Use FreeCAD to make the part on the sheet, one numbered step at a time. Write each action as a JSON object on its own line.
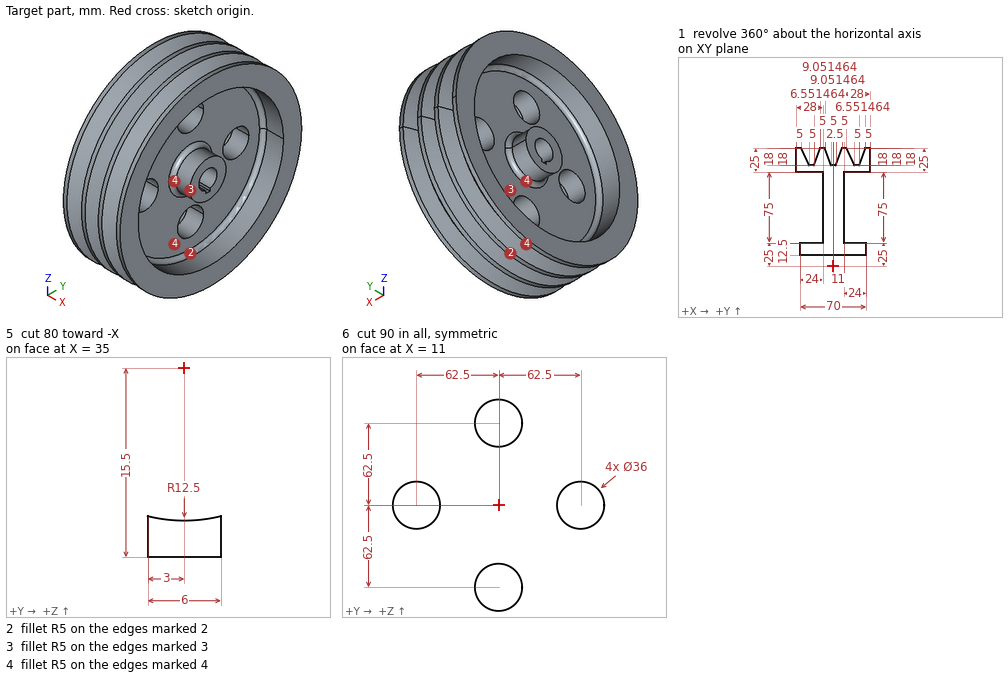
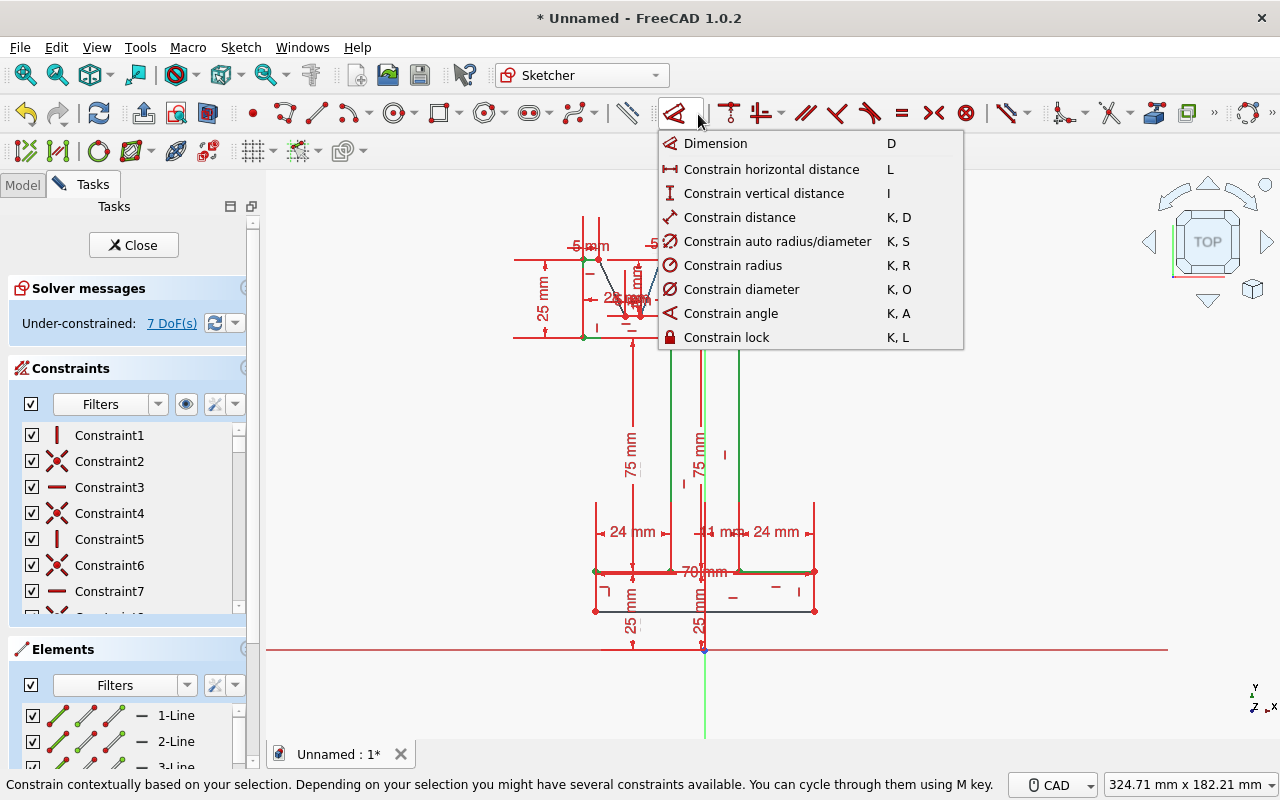
{"action": "left_click", "coordinate": [811, 193]}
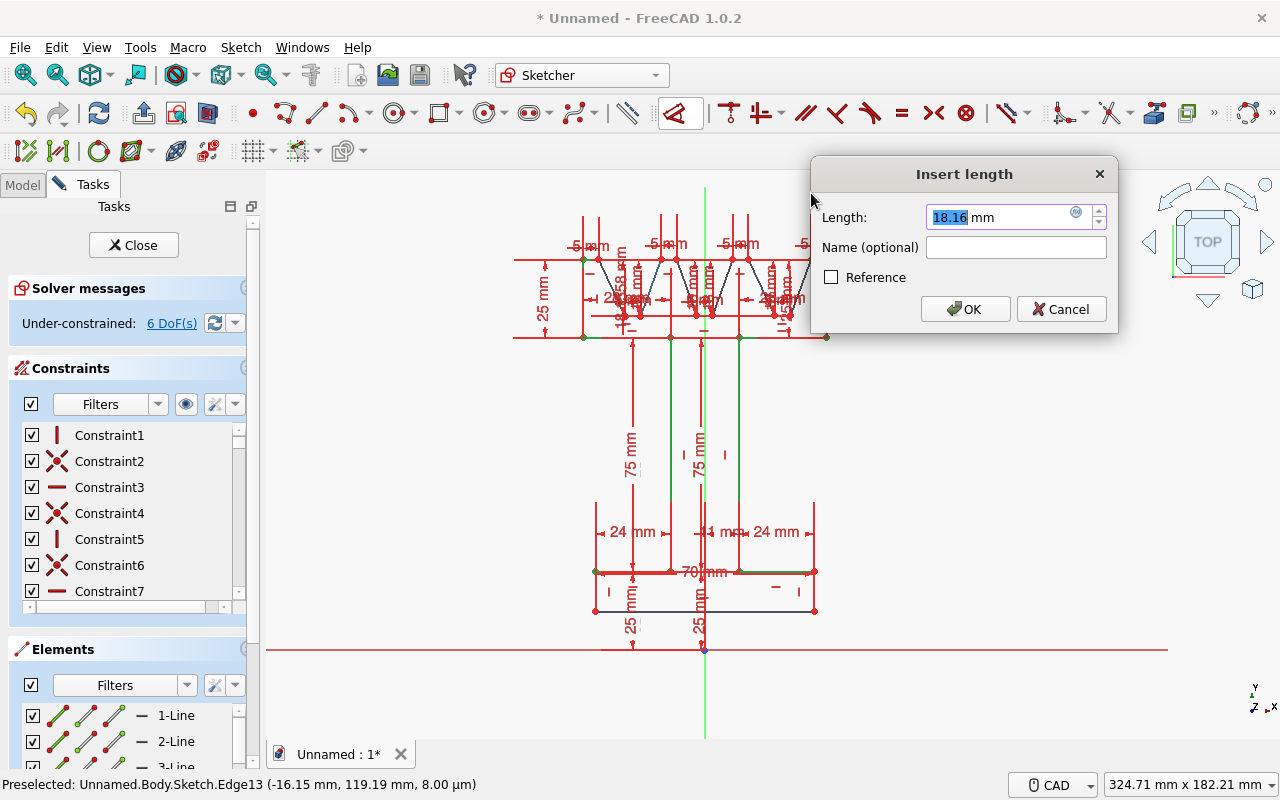
{"action": "type", "text": "18"}
{"action": "key", "text": "Return"}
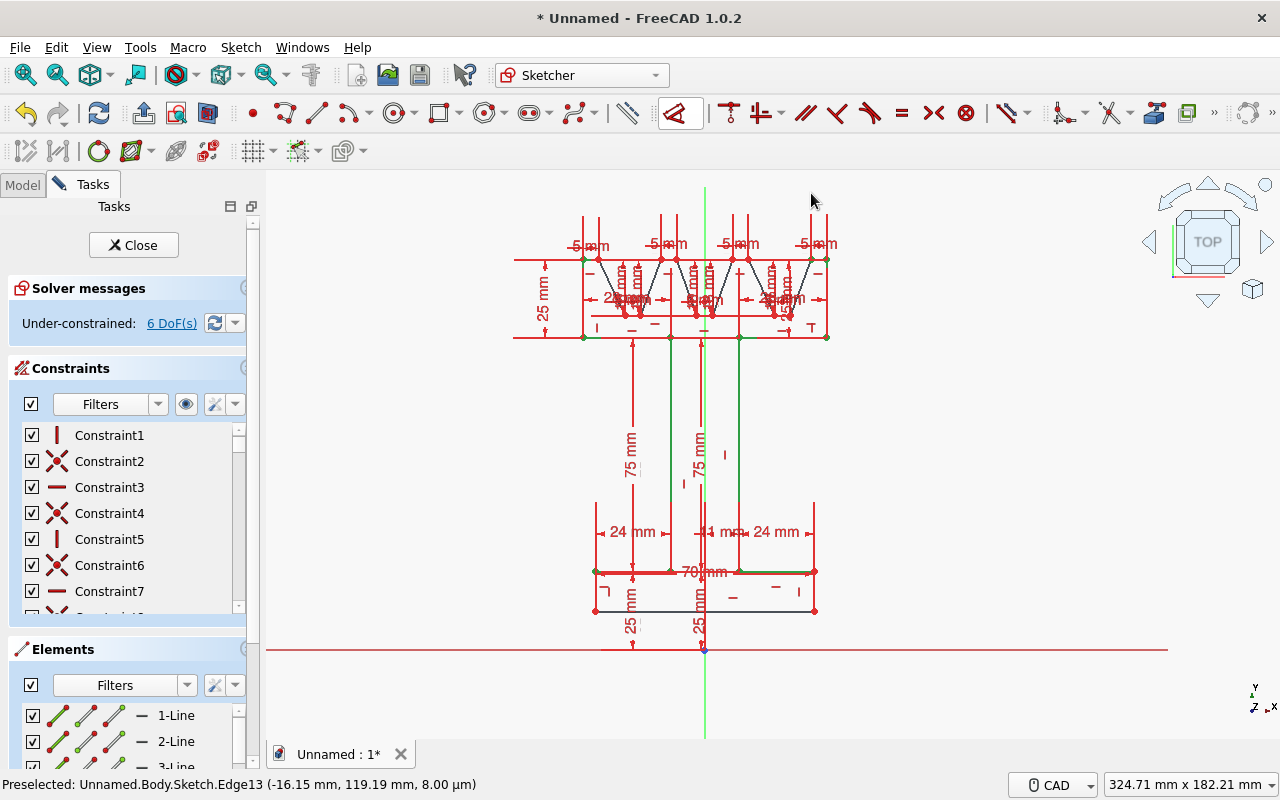
{"action": "left_click", "coordinate": [596, 584]}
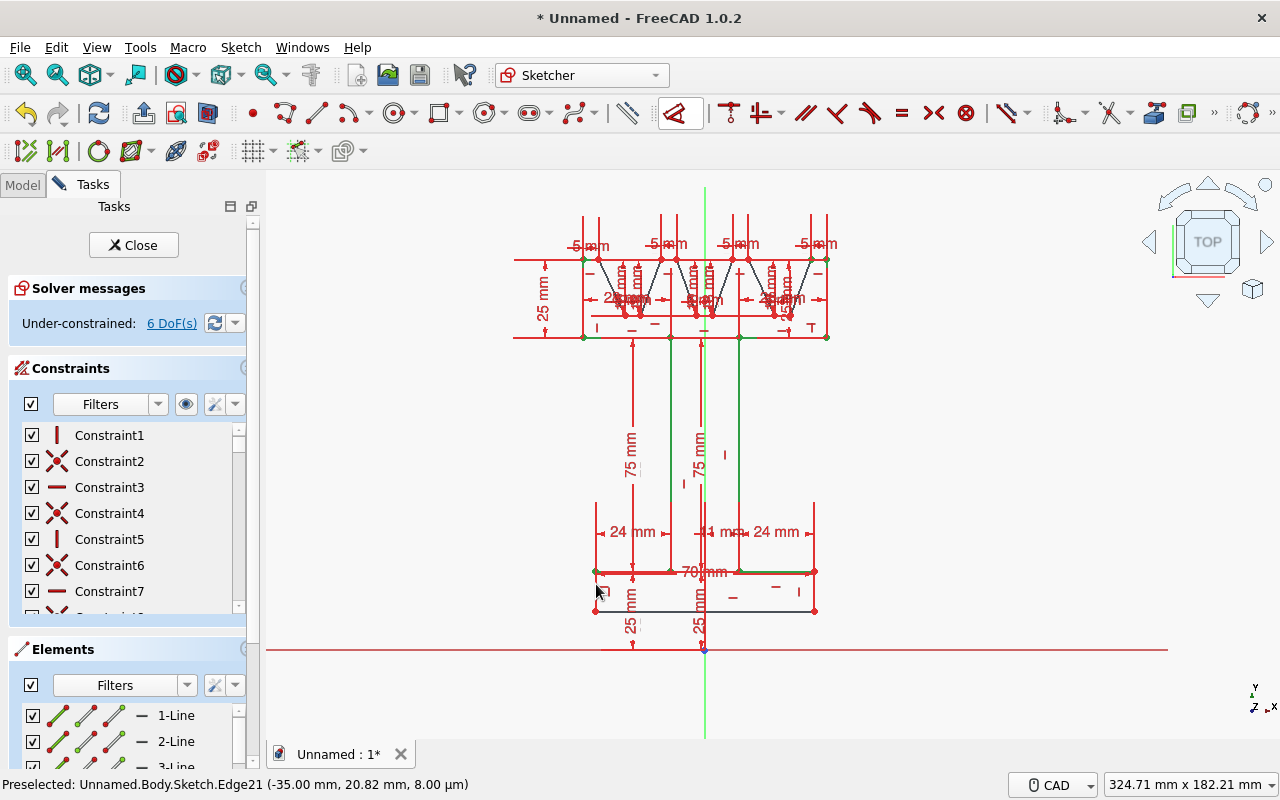
{"action": "key", "text": "i"}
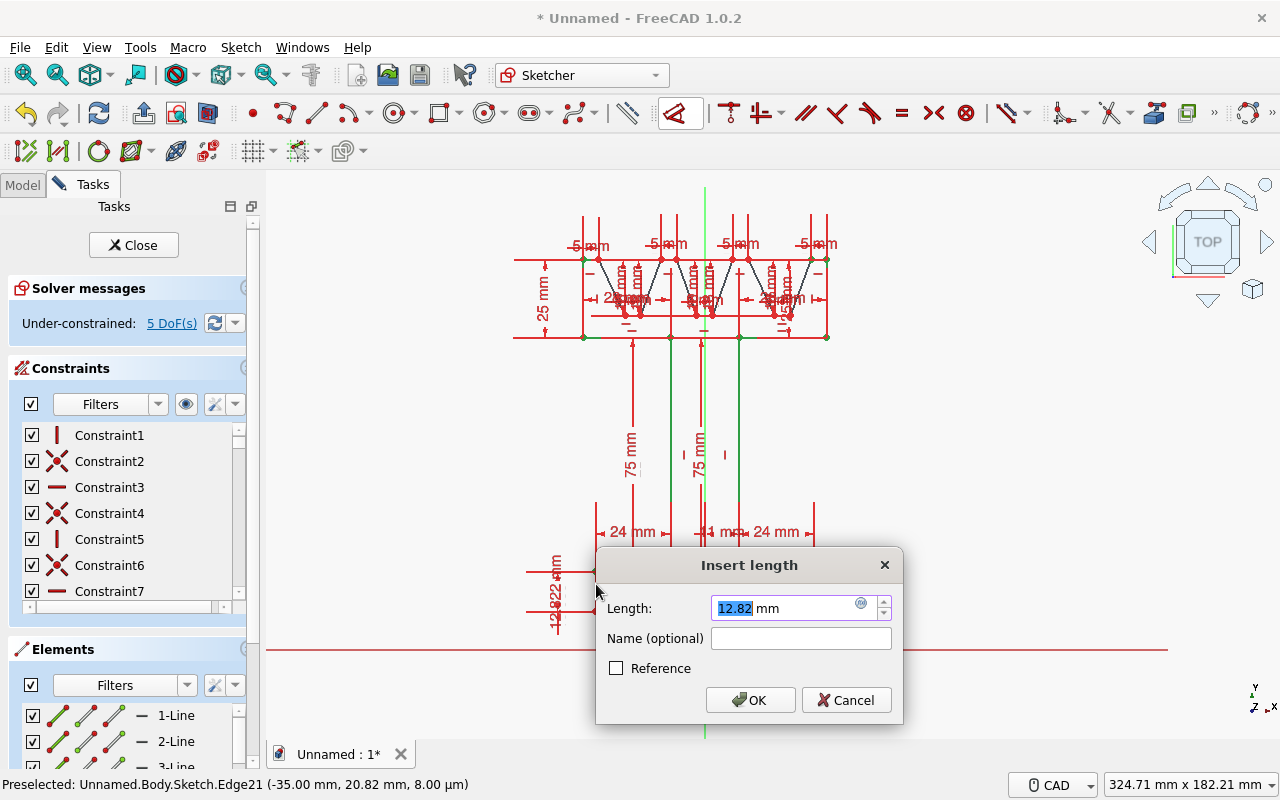
{"action": "type", "text": "12.5"}
{"action": "key", "text": "Return"}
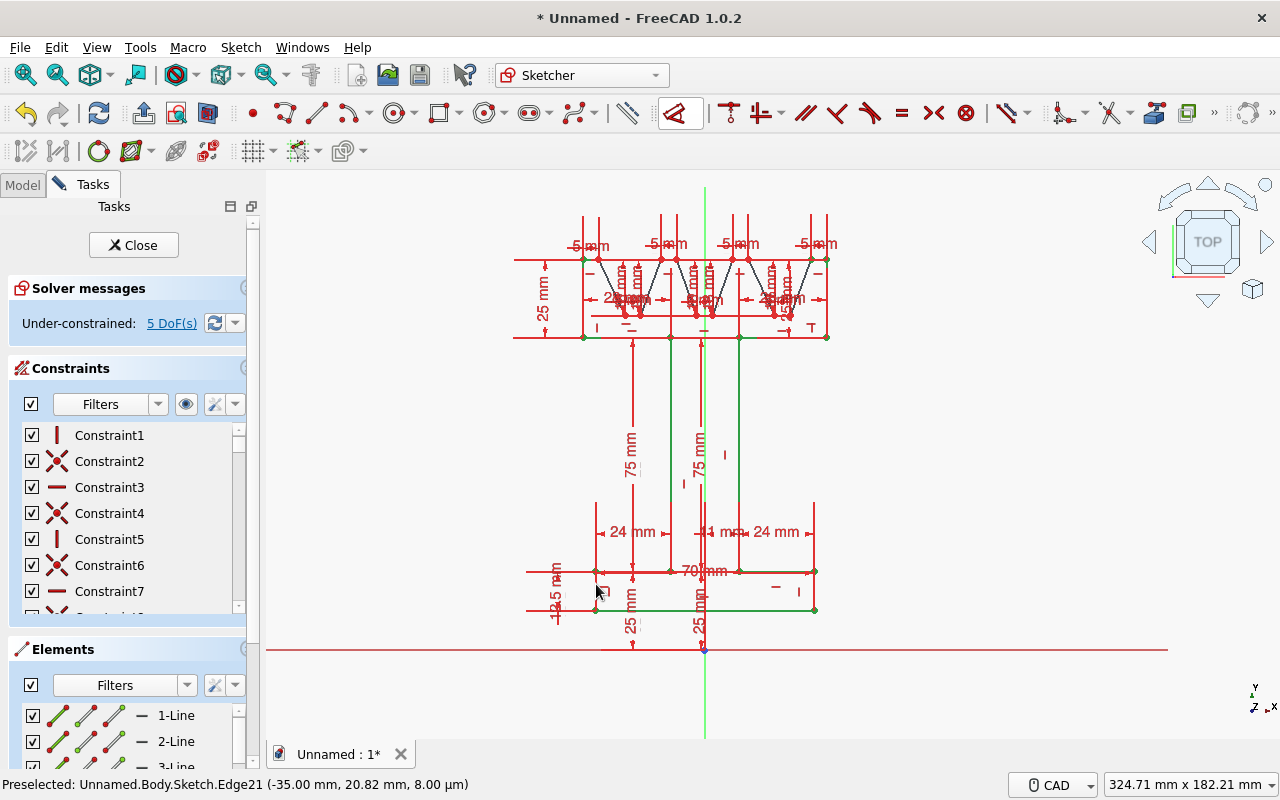
{"action": "scroll", "coordinate": [713, 316], "scroll_direction": "up", "scroll_amount": 9}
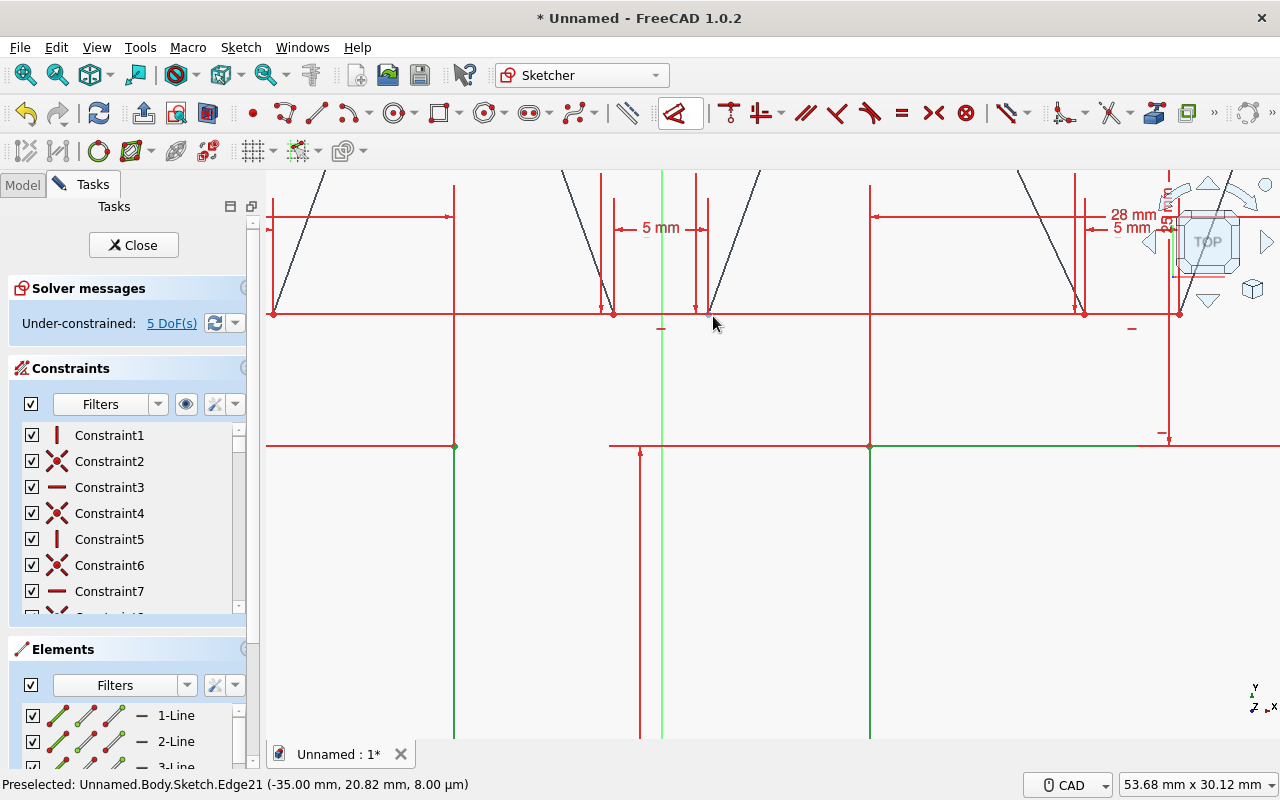
{"action": "left_click", "coordinate": [708, 314]}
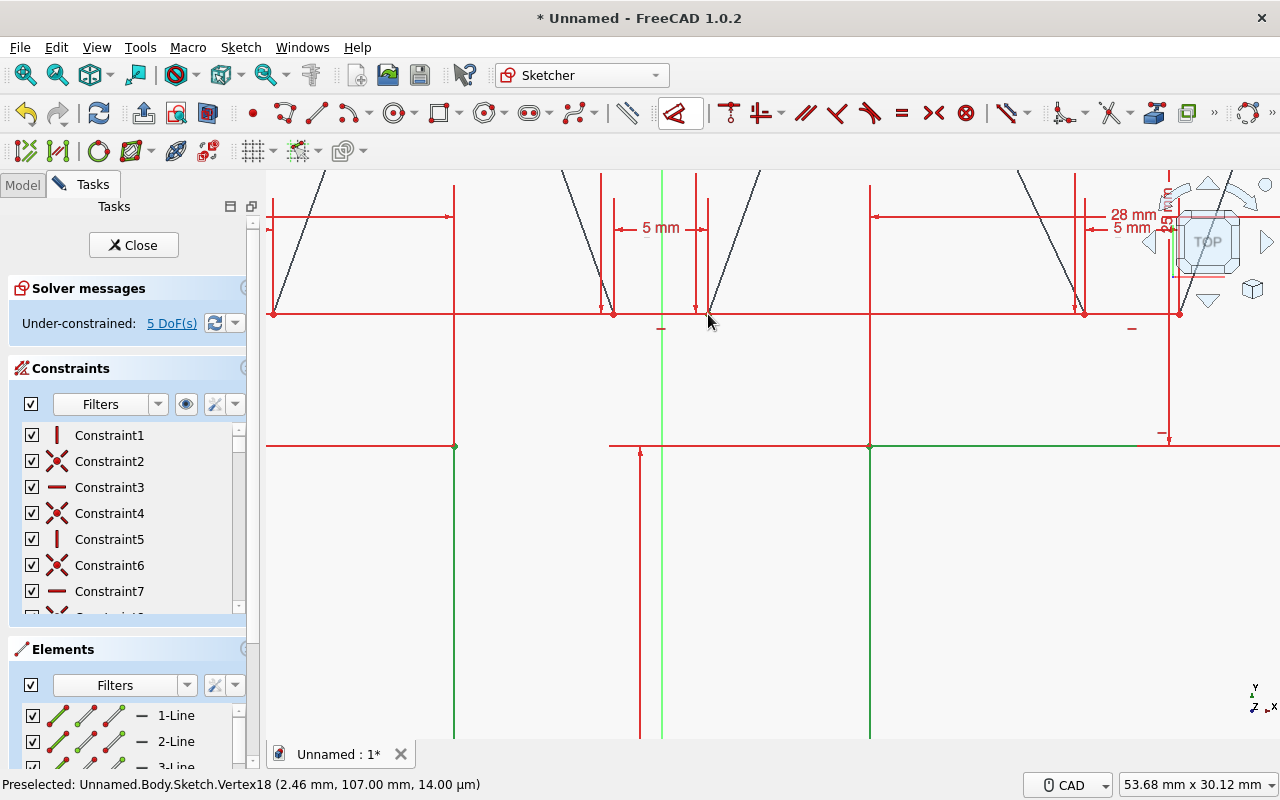
{"action": "left_click", "coordinate": [698, 114]}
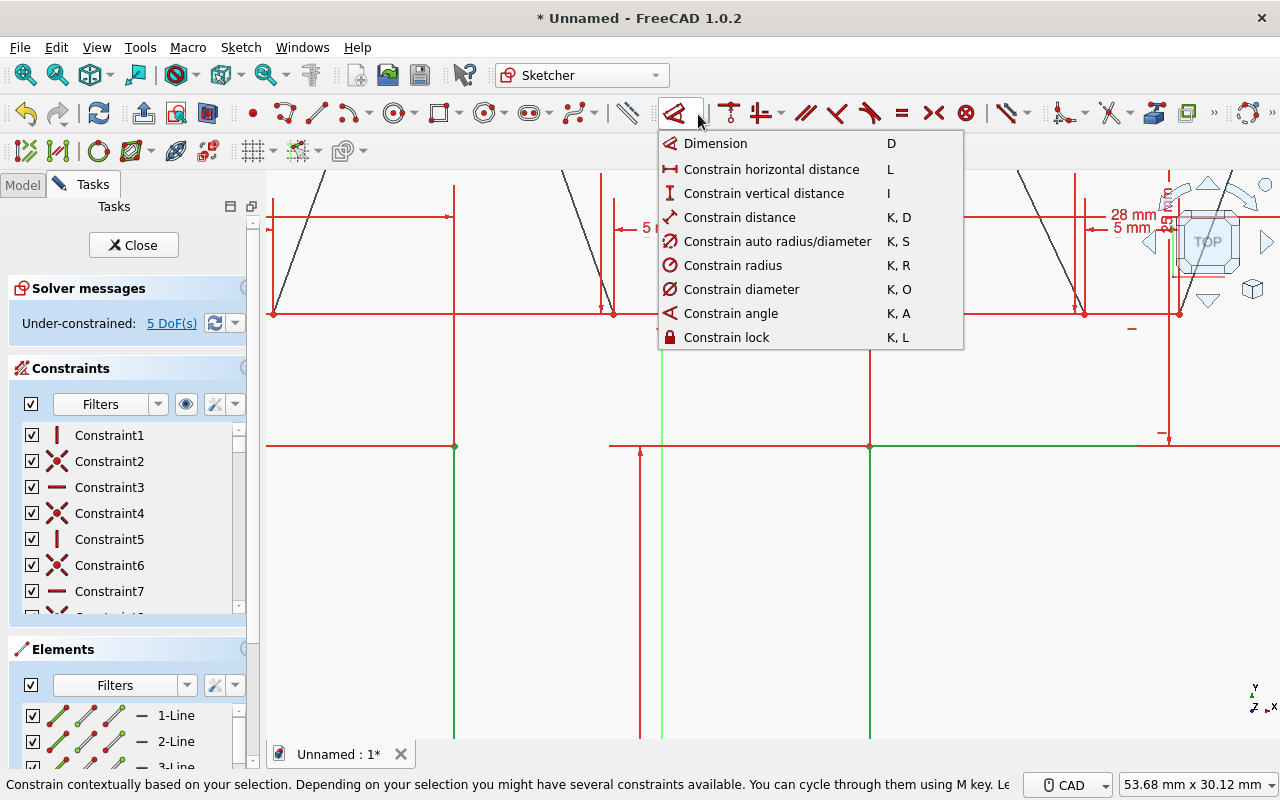
{"action": "left_click", "coordinate": [811, 169]}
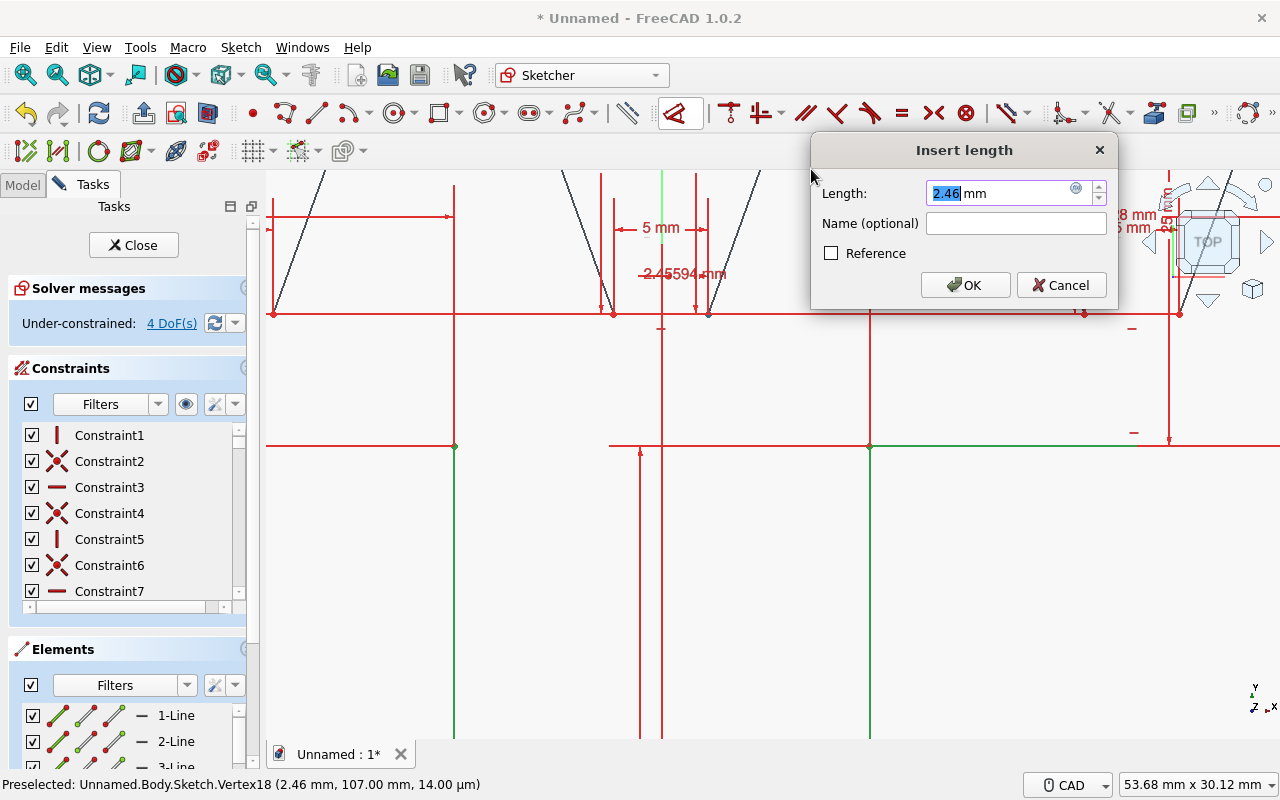
{"action": "type", "text": "2.5"}
{"action": "key", "text": "Return"}